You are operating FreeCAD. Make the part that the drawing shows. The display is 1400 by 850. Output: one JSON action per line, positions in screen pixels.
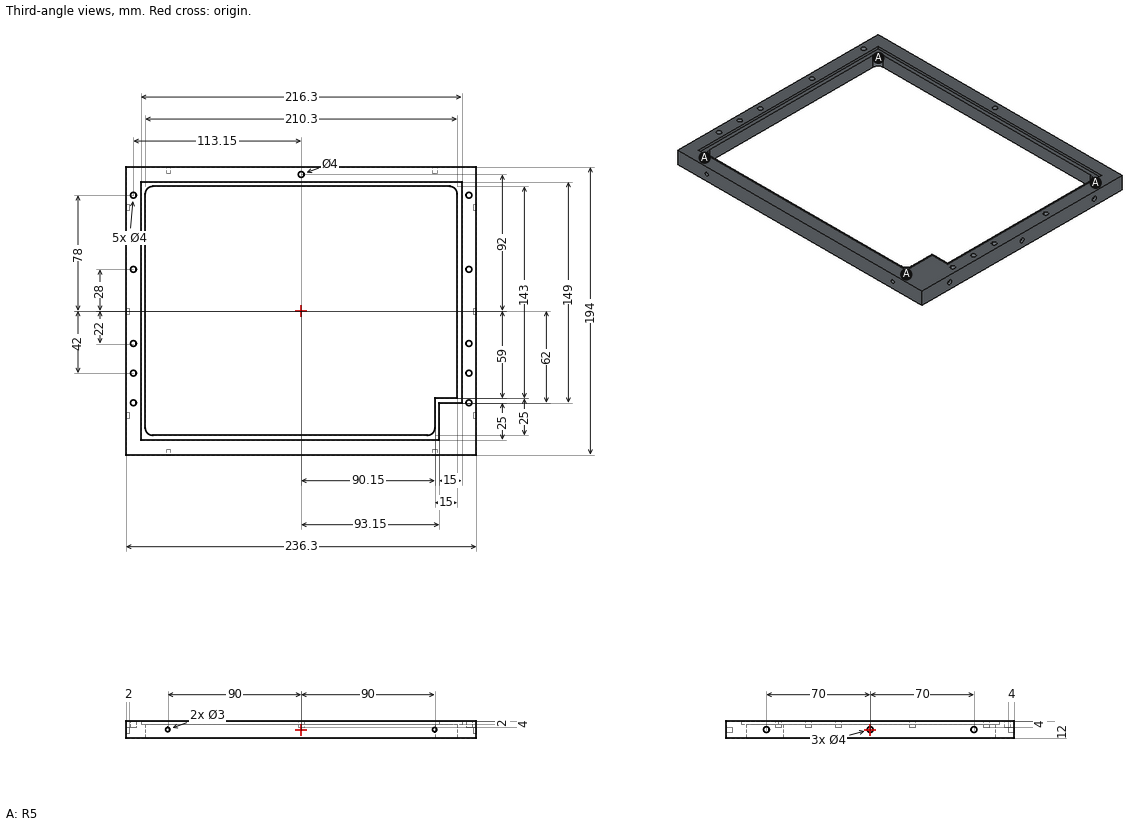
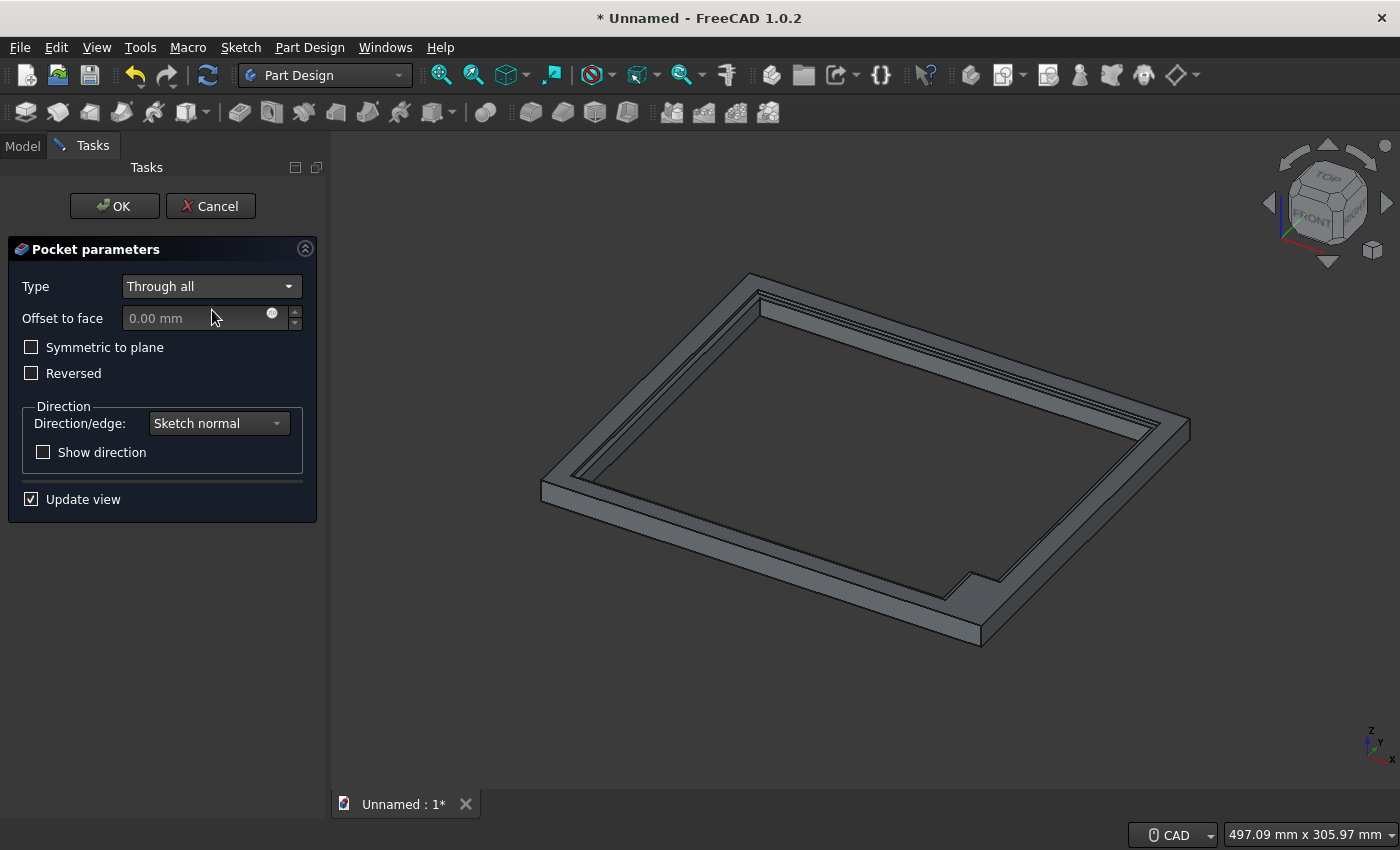
{"action": "left_click", "coordinate": [115, 206]}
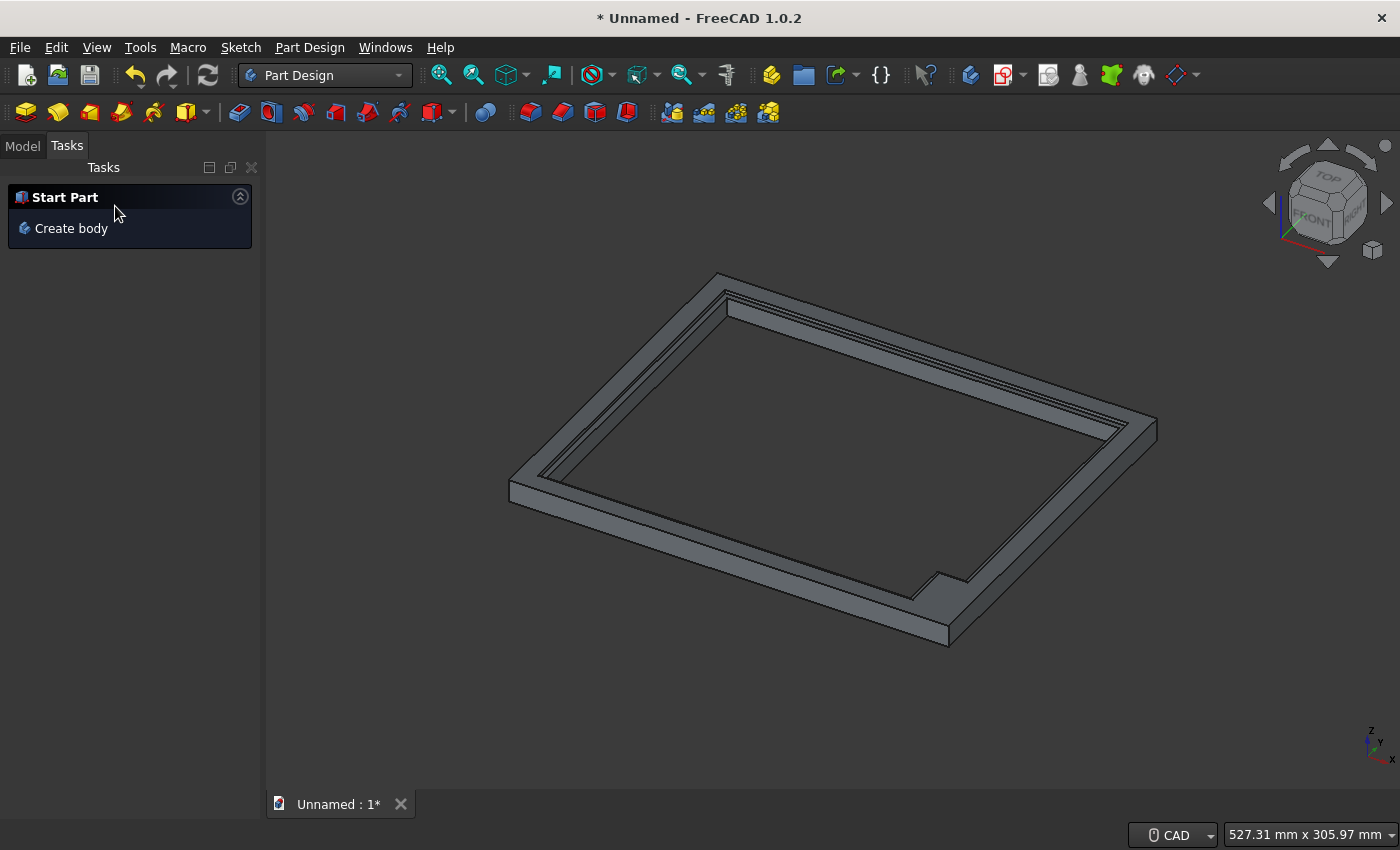
{"action": "scroll", "coordinate": [911, 606], "scroll_direction": "up", "scroll_amount": 4}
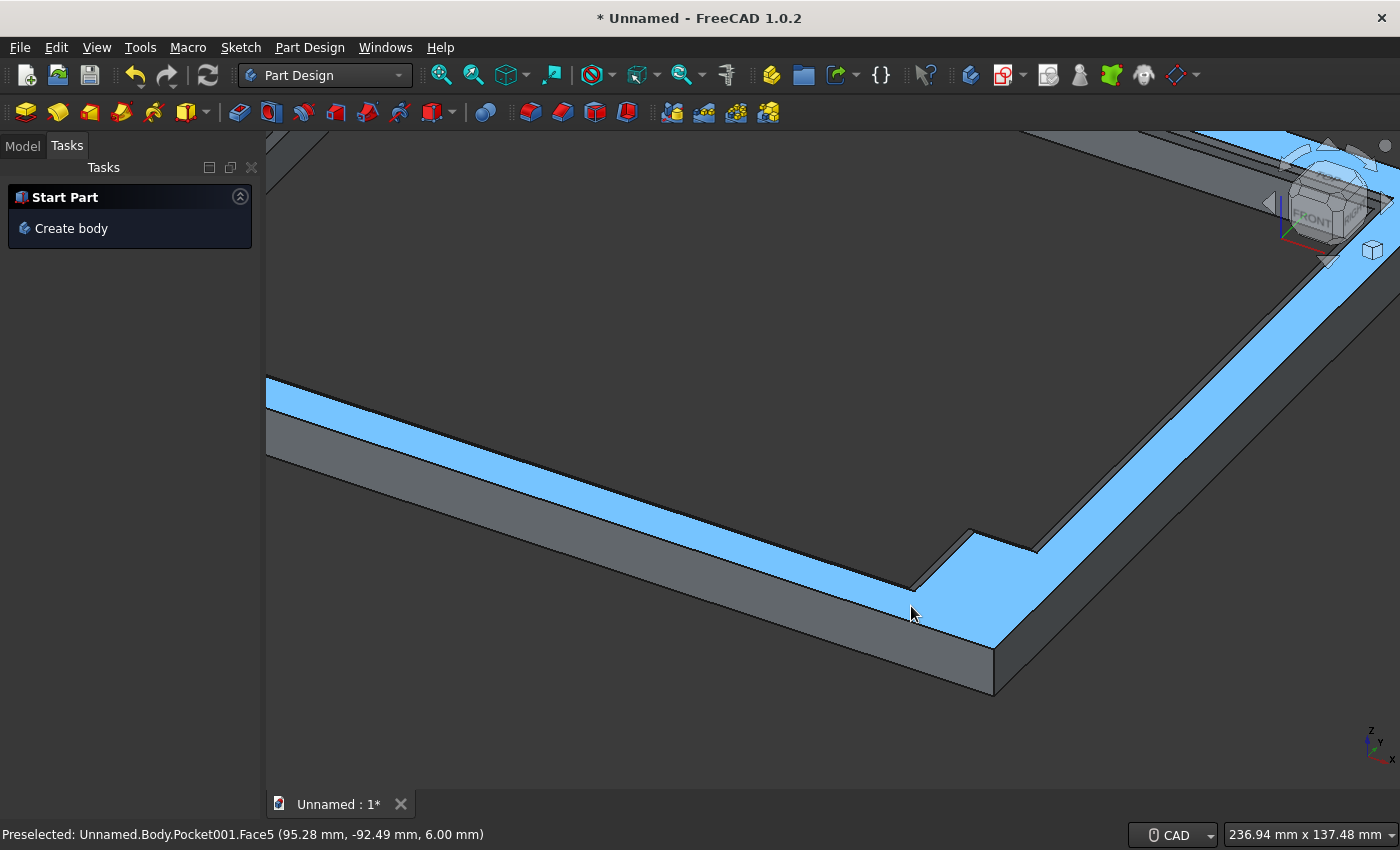
{"action": "left_click", "coordinate": [442, 76]}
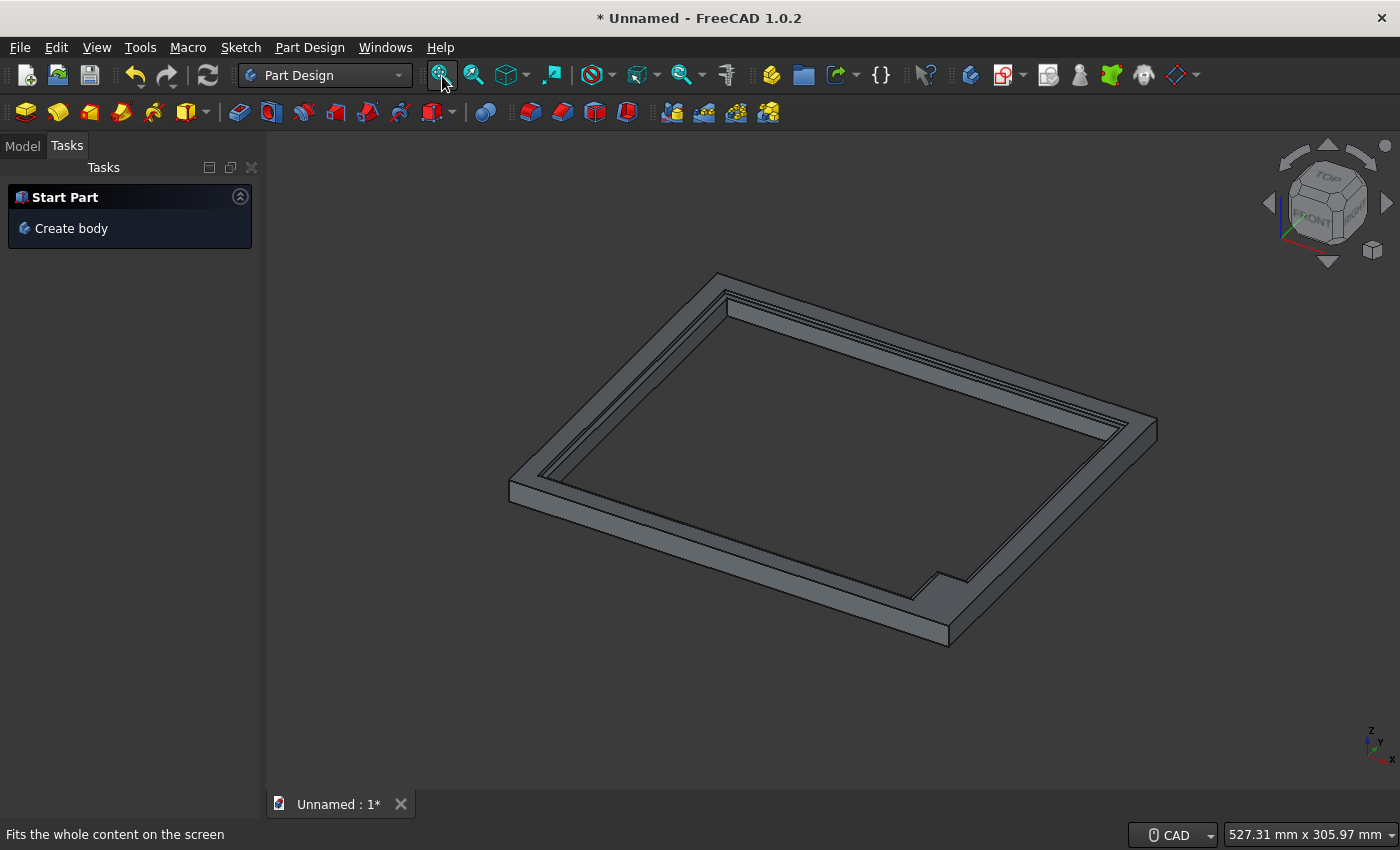
{"action": "key", "text": "0"}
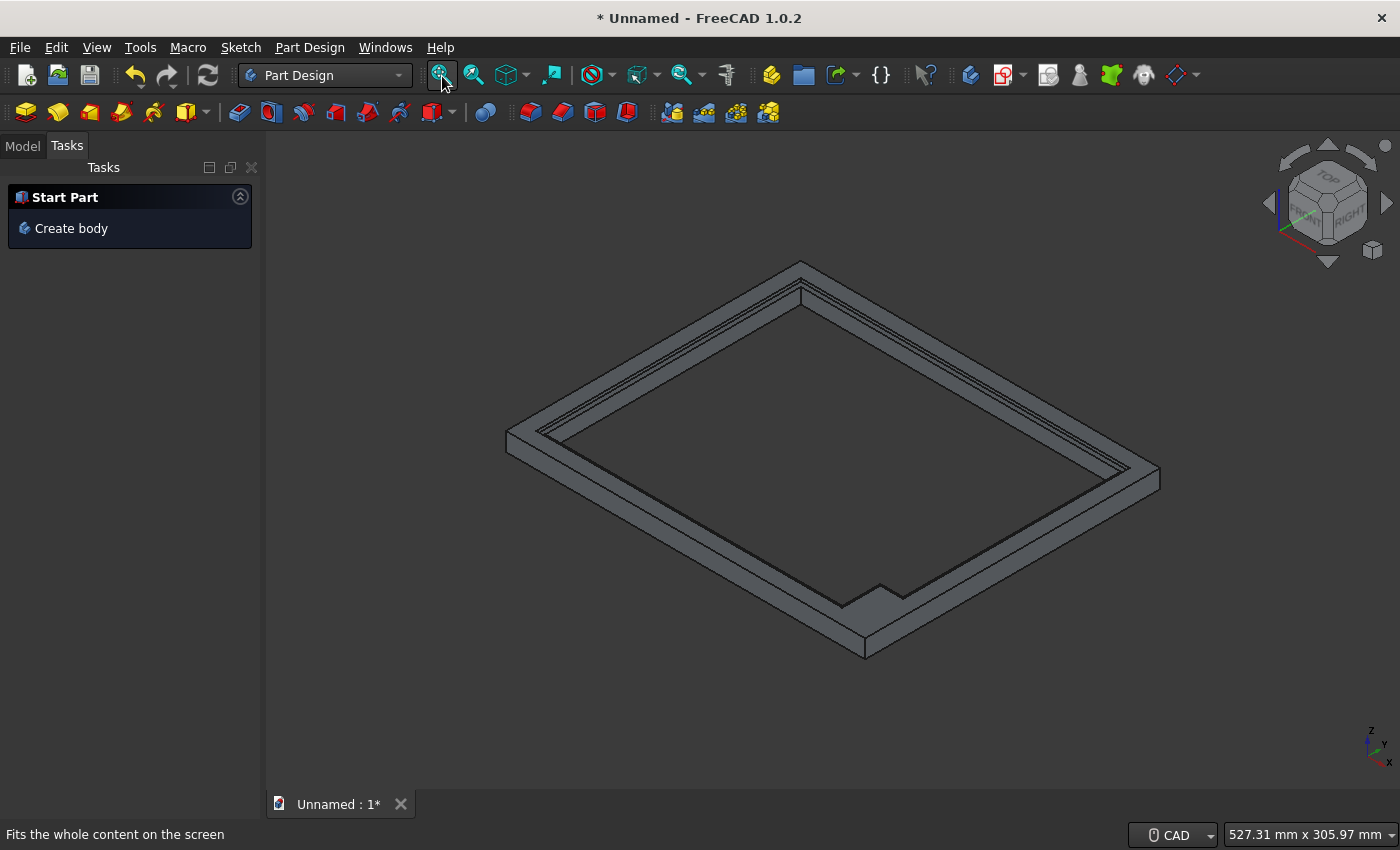
{"action": "scroll", "coordinate": [842, 614], "scroll_direction": "up", "scroll_amount": 4}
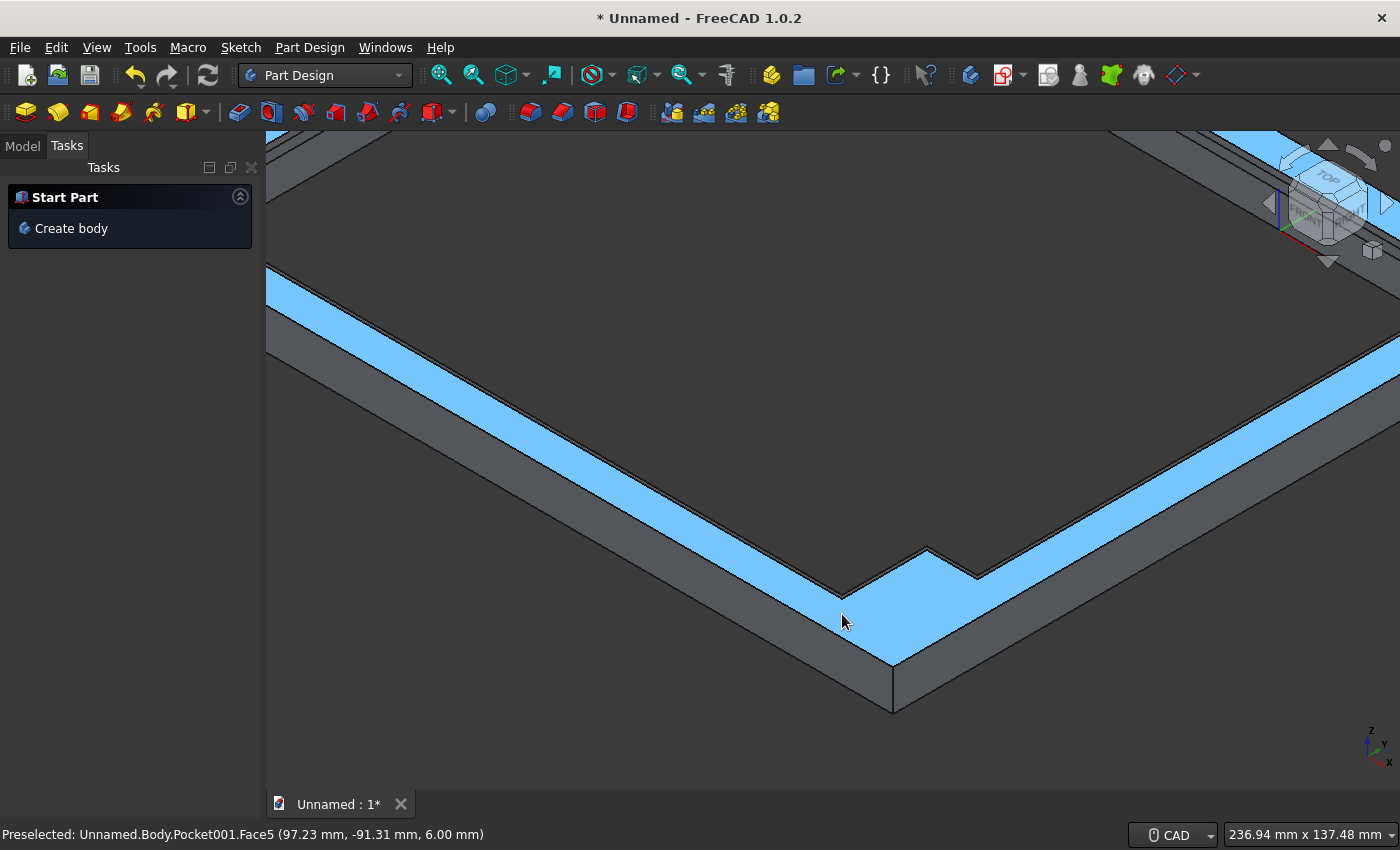
{"action": "left_click", "coordinate": [442, 76]}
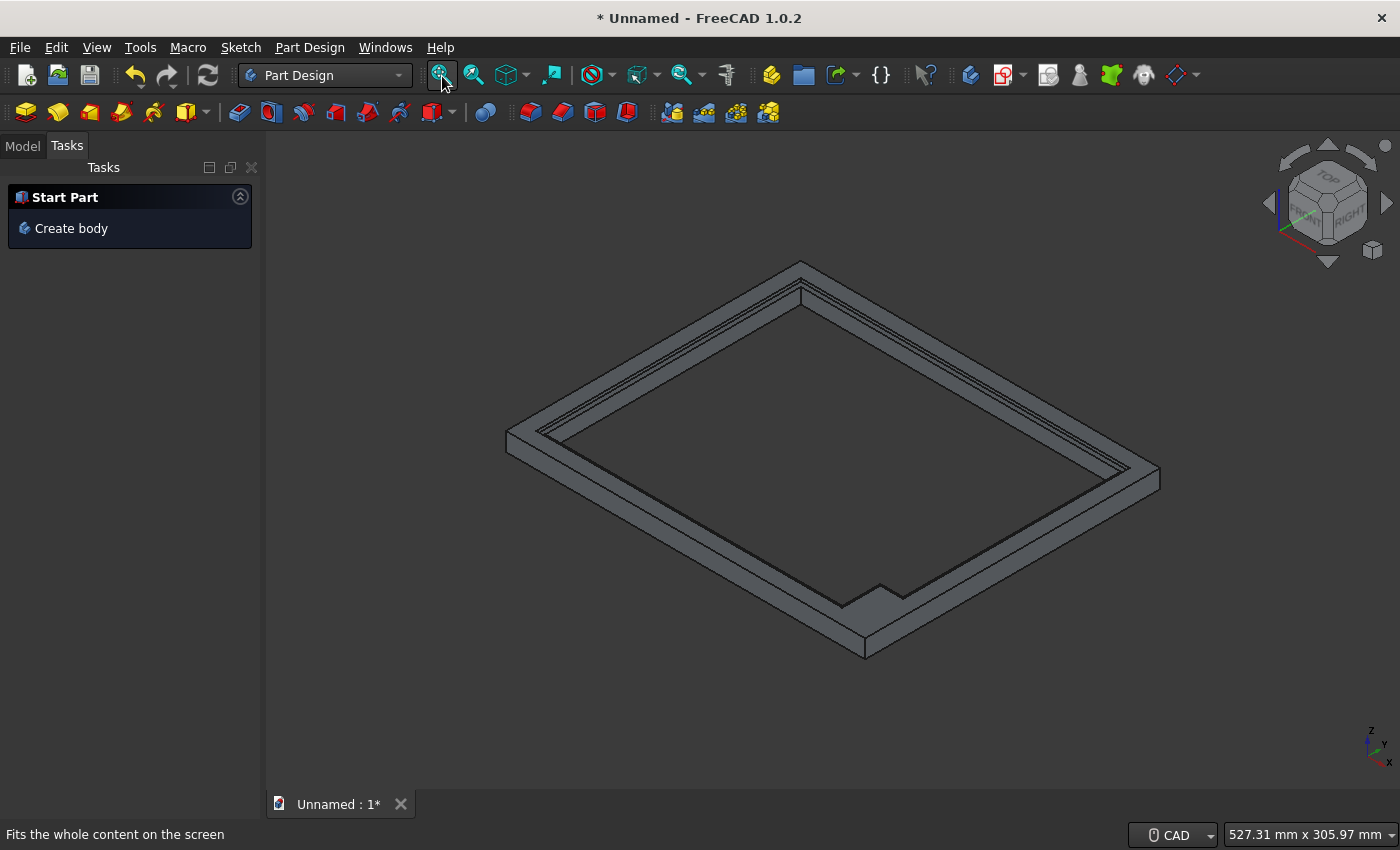
{"action": "key", "text": "2"}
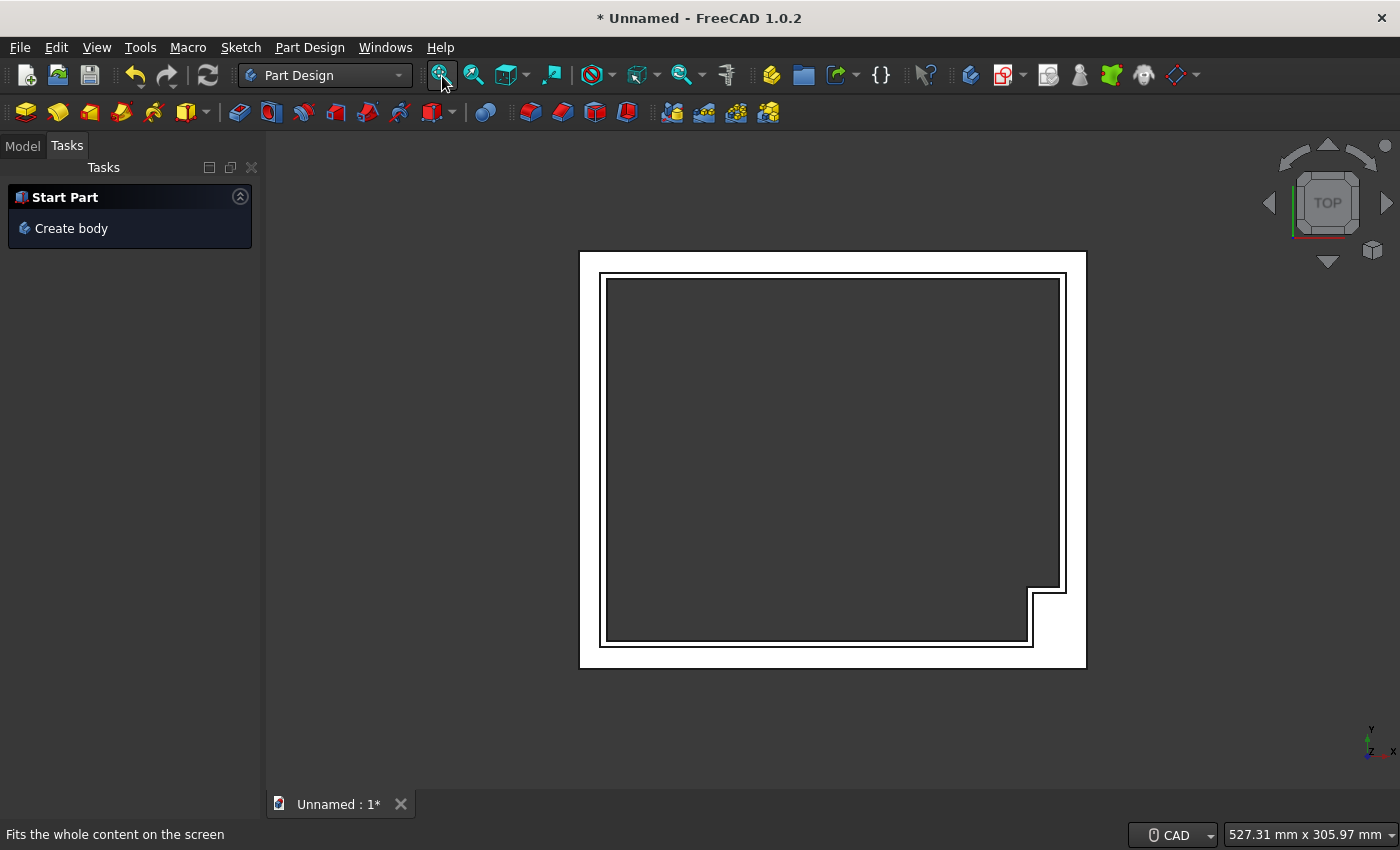
{"action": "scroll", "coordinate": [1027, 640], "scroll_direction": "up", "scroll_amount": 4}